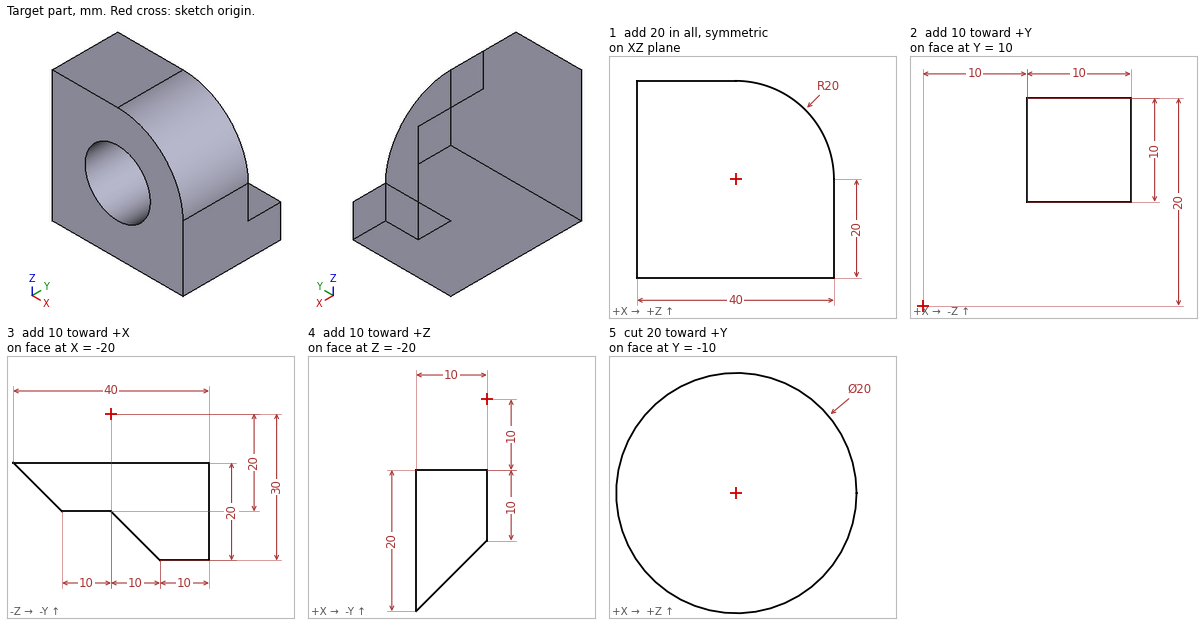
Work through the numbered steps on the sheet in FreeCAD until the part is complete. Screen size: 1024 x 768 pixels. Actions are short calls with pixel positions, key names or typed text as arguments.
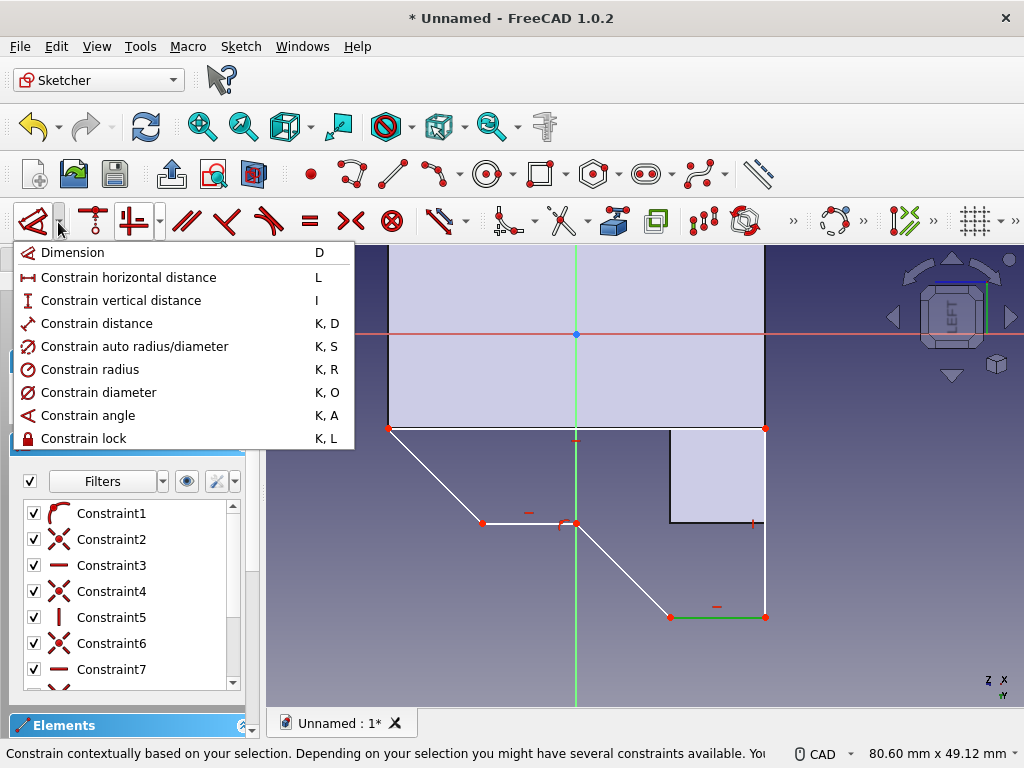
click(184, 278)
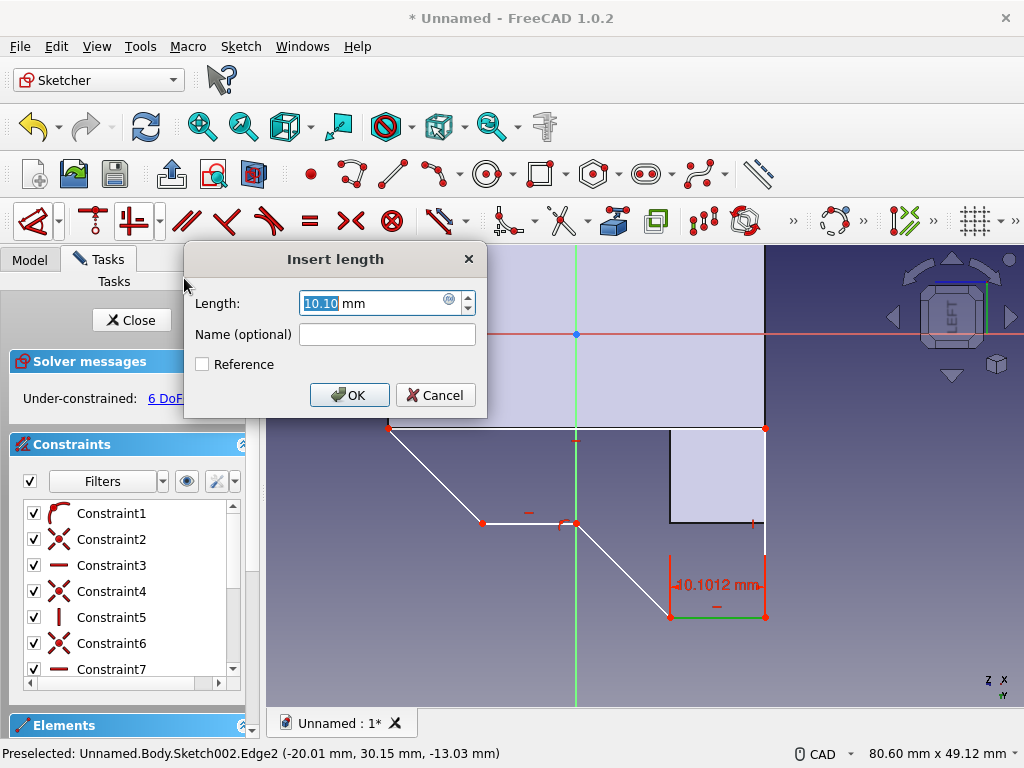
text(10)
key(Return)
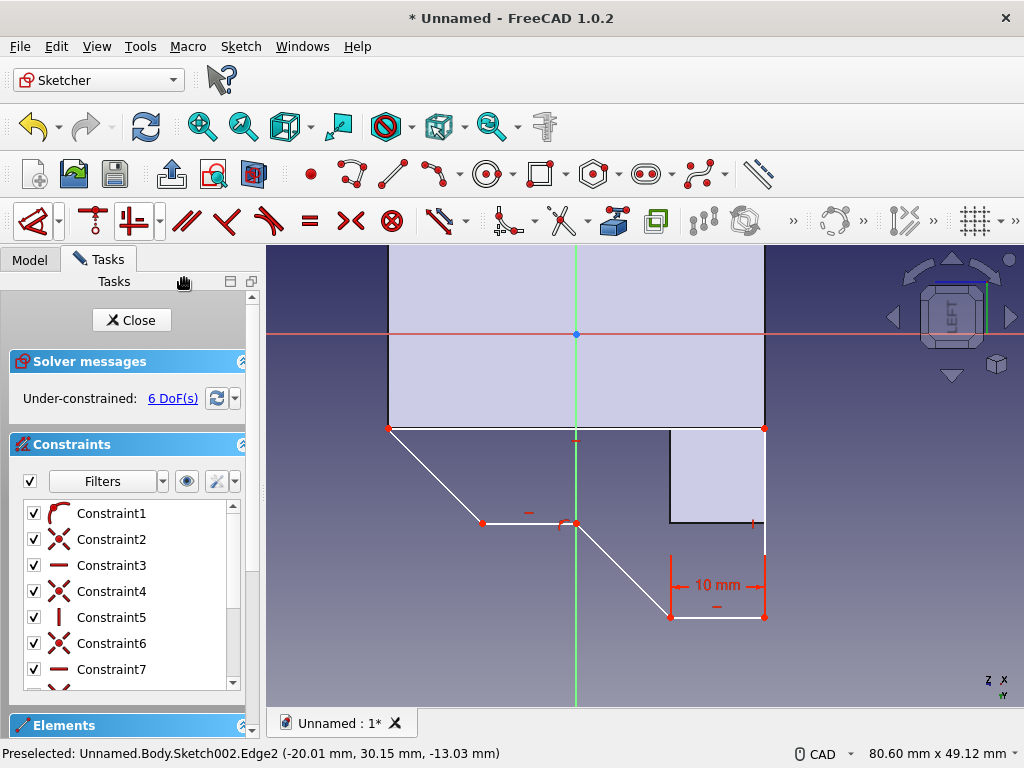
click(765, 561)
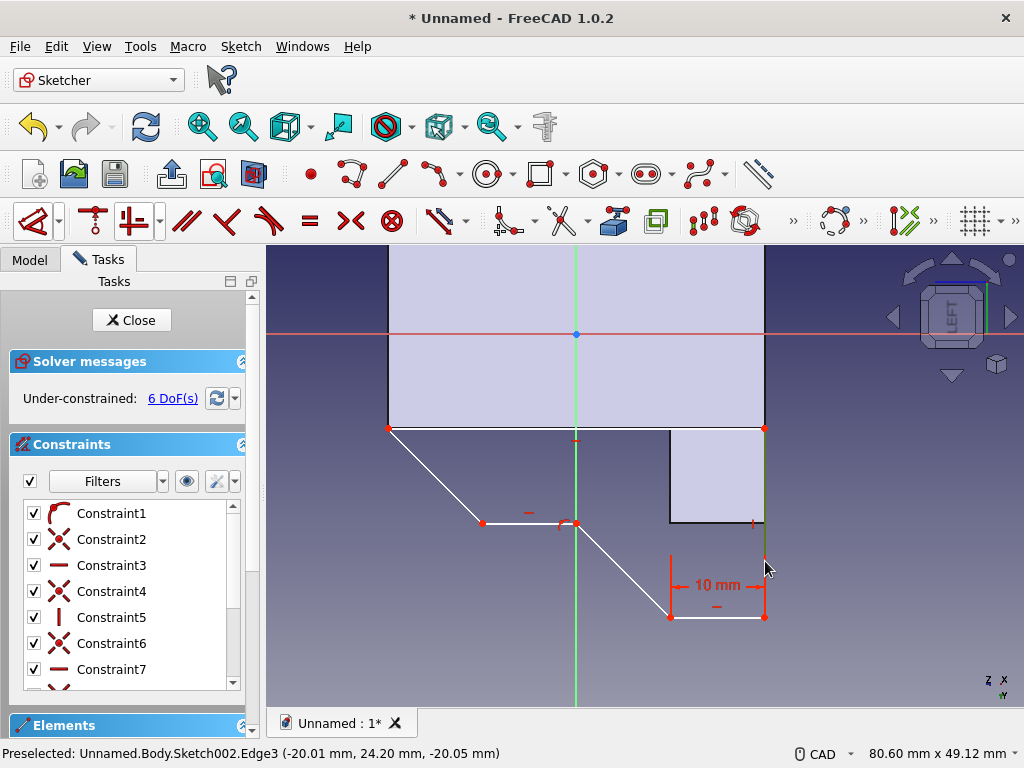
key(i)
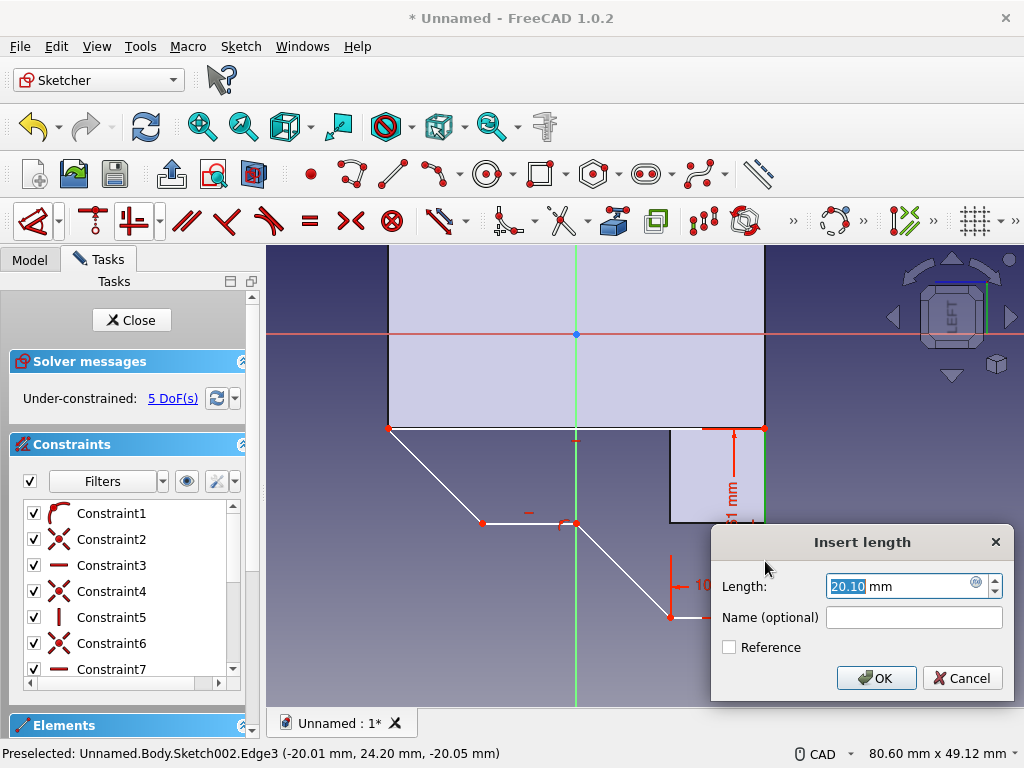
text(20)
key(Return)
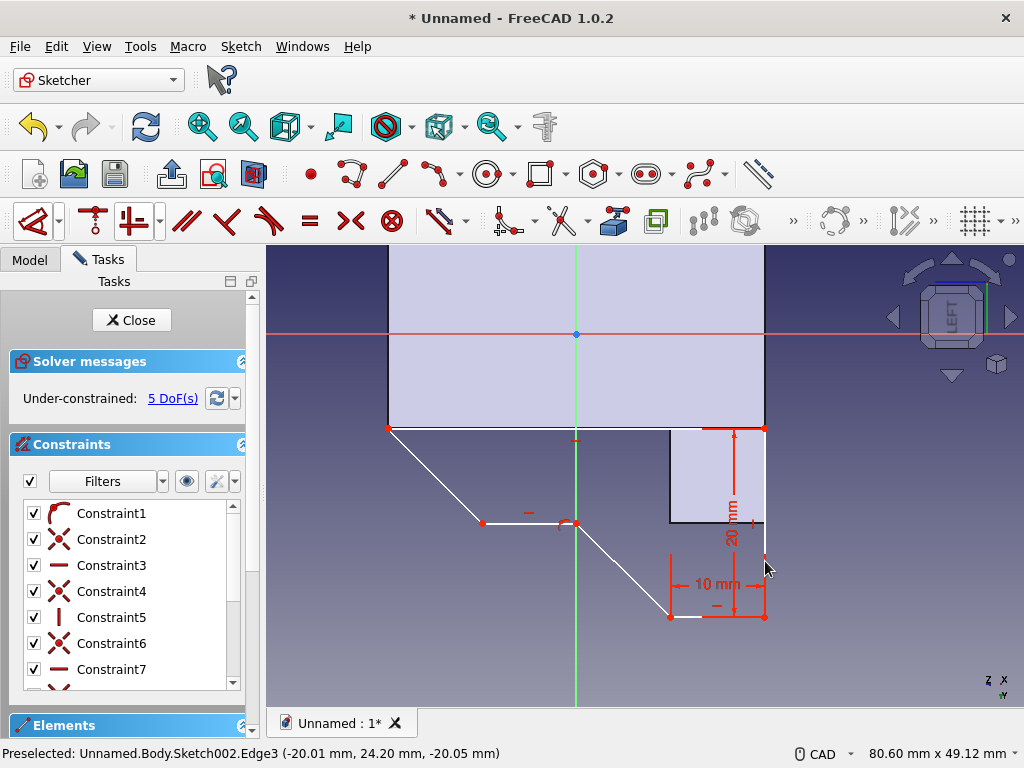
click(652, 429)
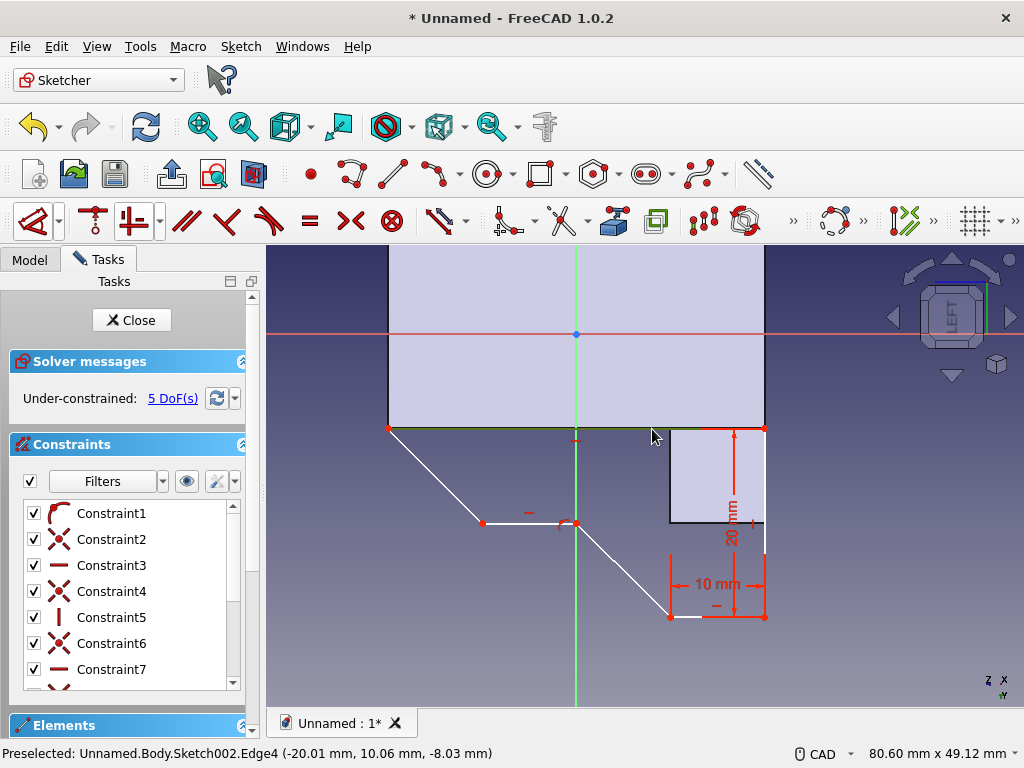
key(l)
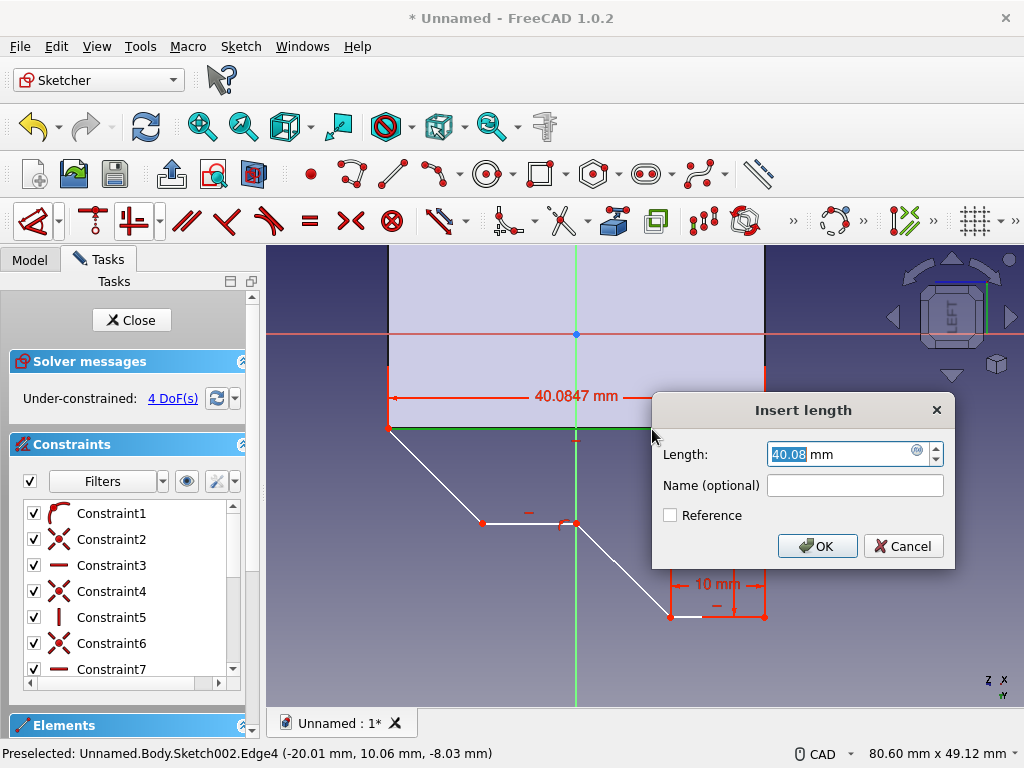
text(40)
key(Return)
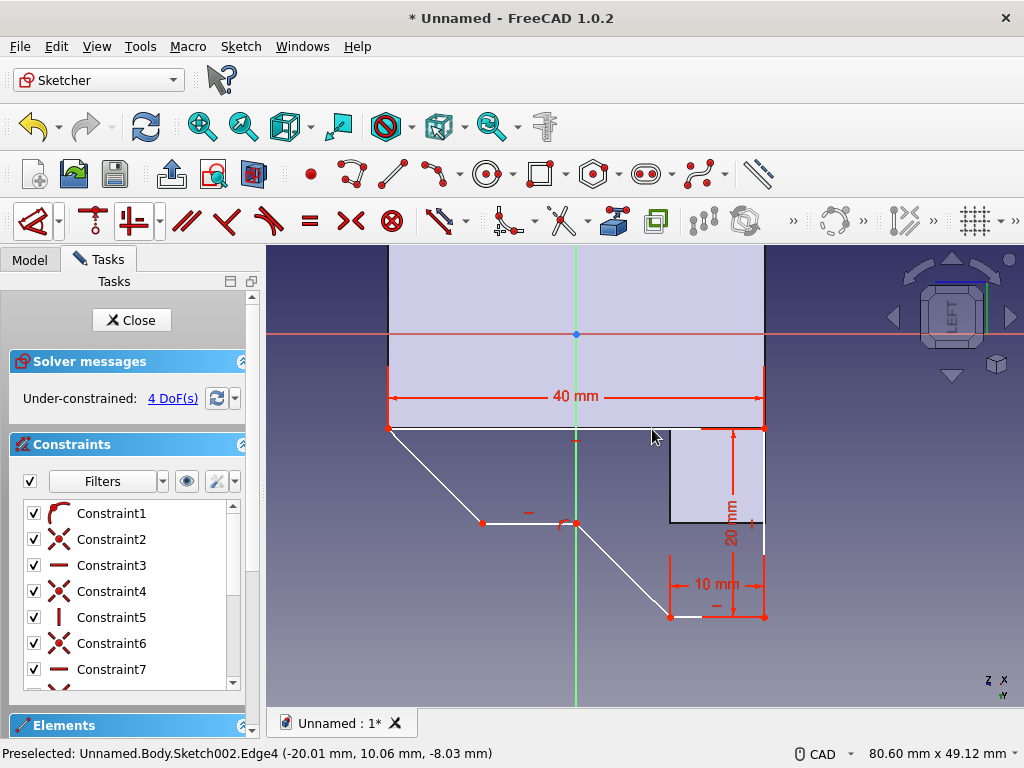
click(510, 524)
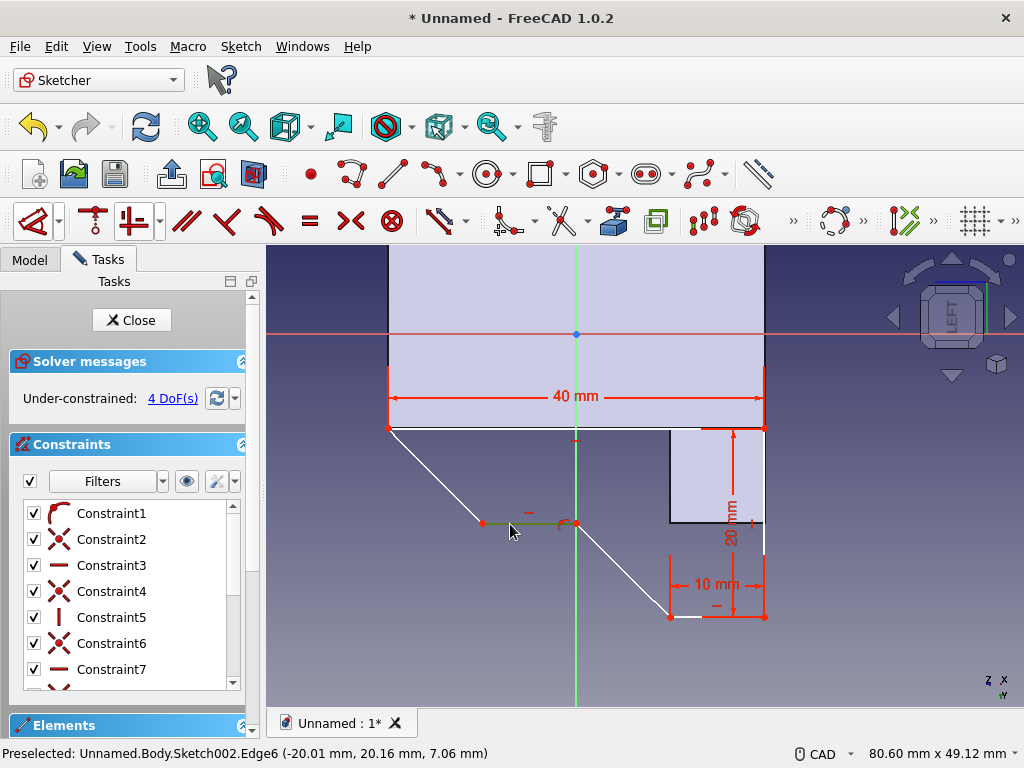
click(58, 222)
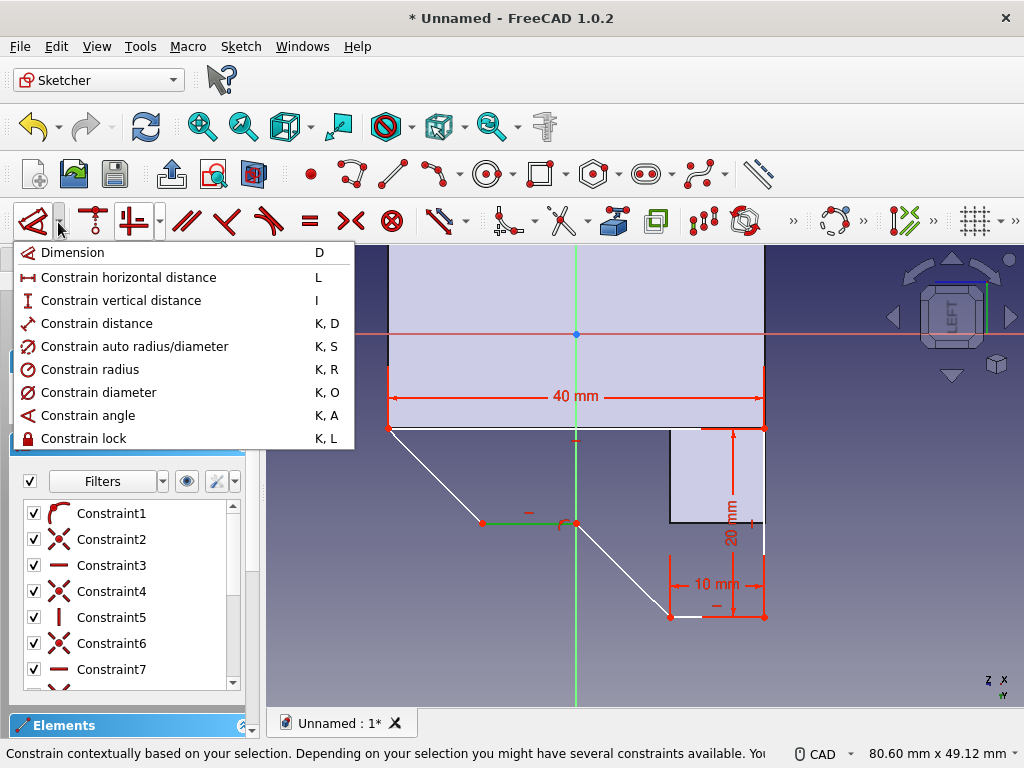
click(184, 278)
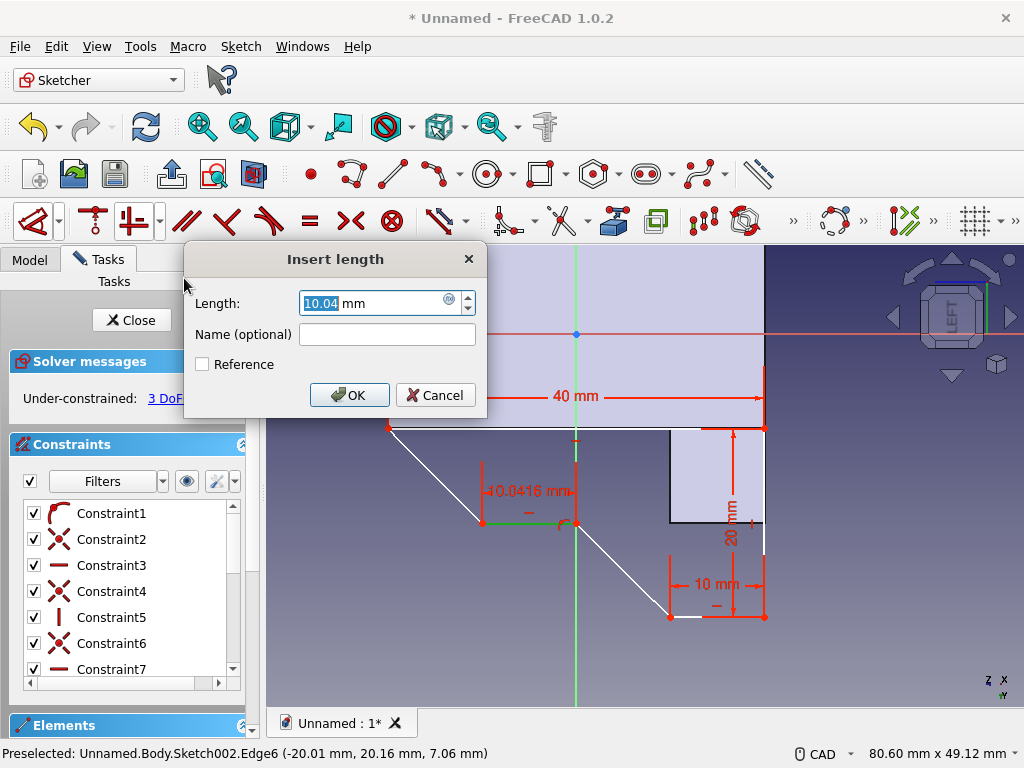
text(10)
key(Return)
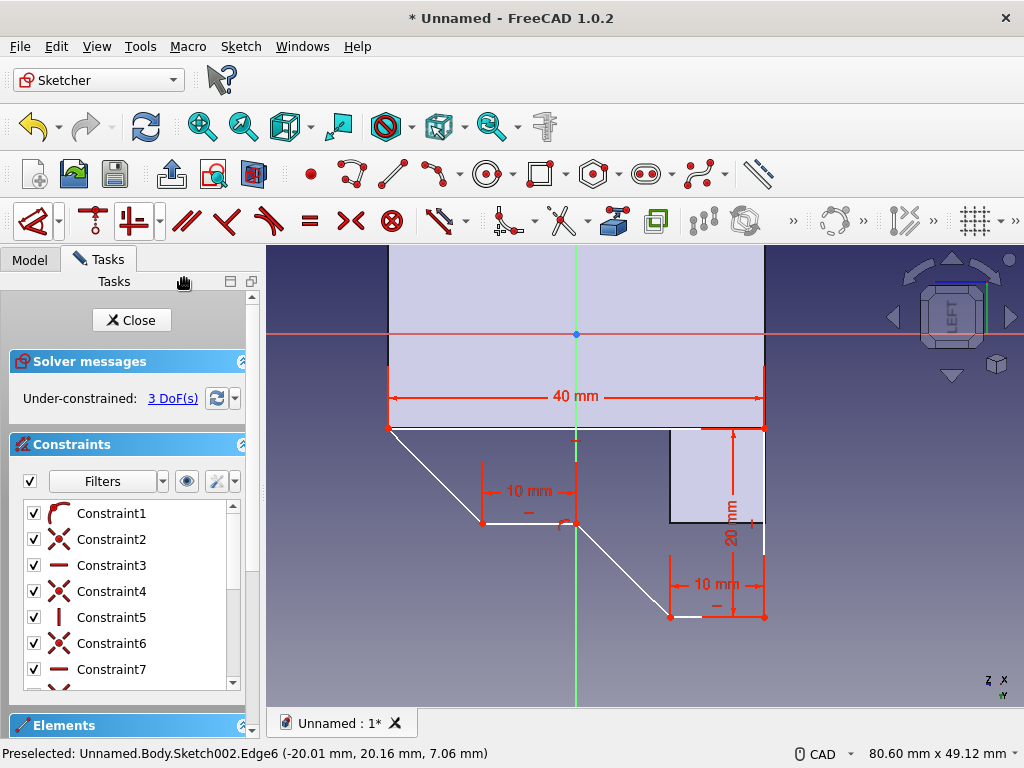
click(576, 524)